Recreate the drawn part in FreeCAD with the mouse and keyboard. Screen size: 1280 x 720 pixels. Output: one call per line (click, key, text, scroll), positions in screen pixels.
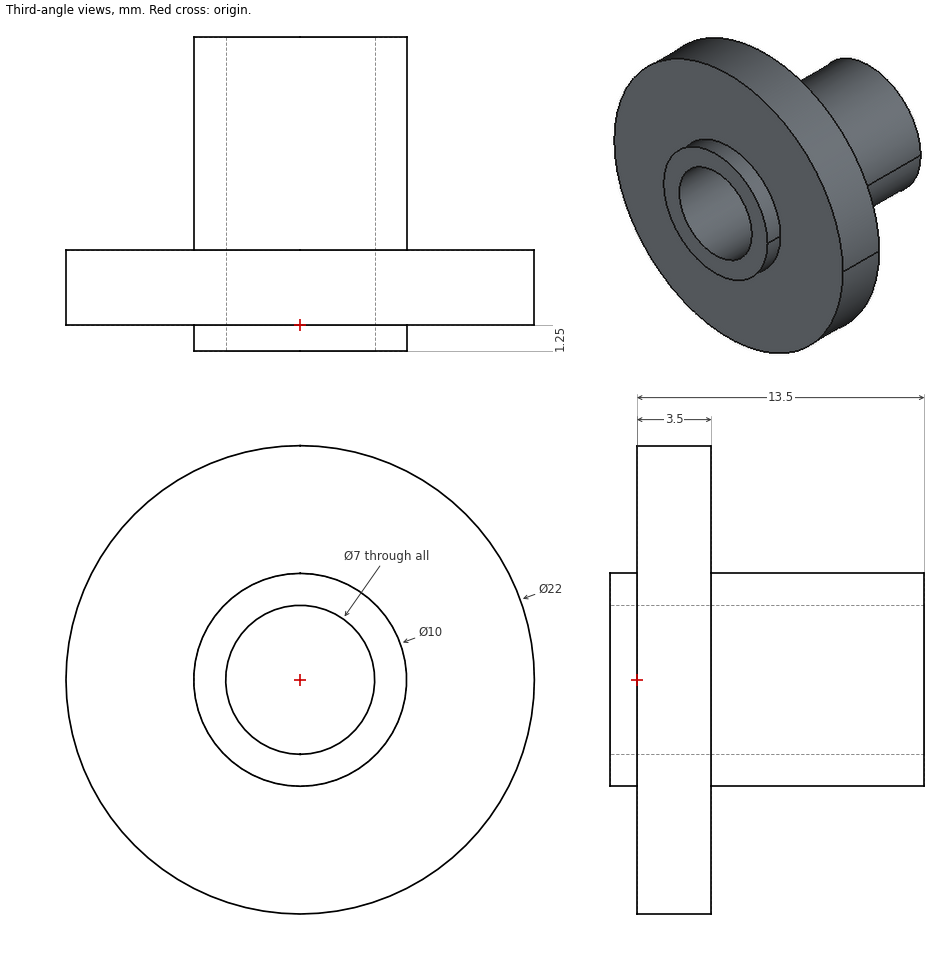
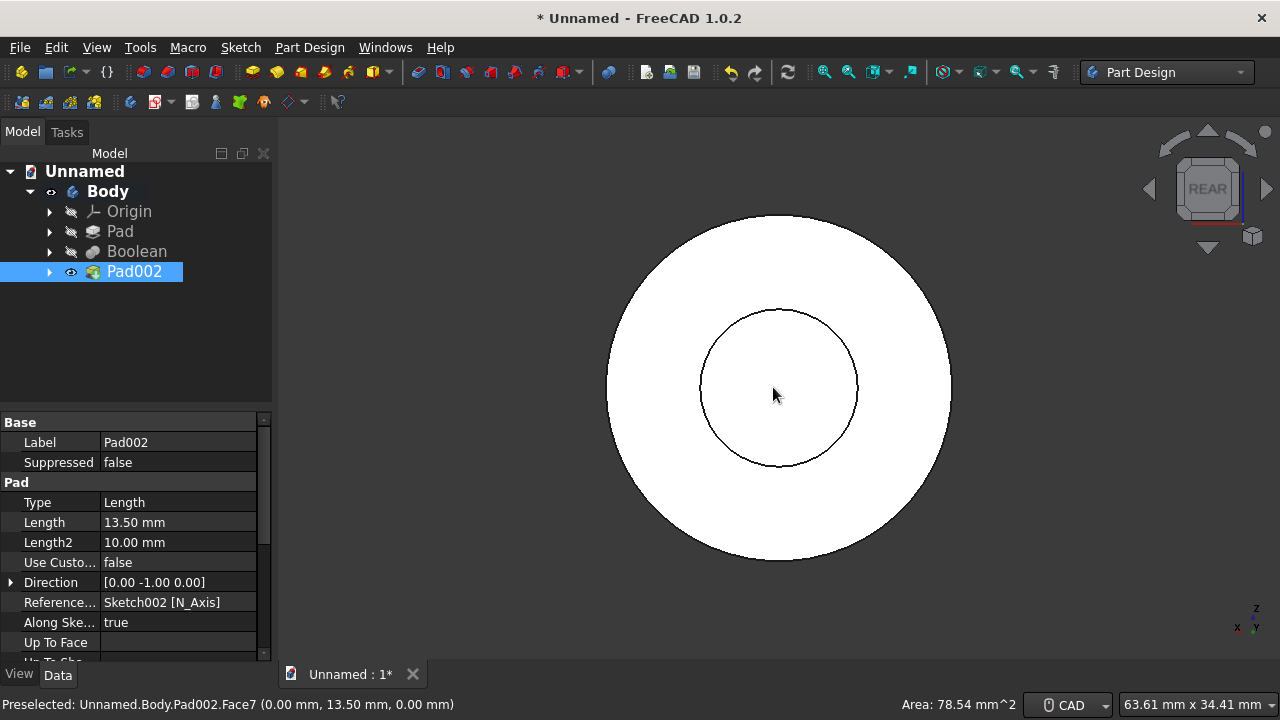
click(156, 102)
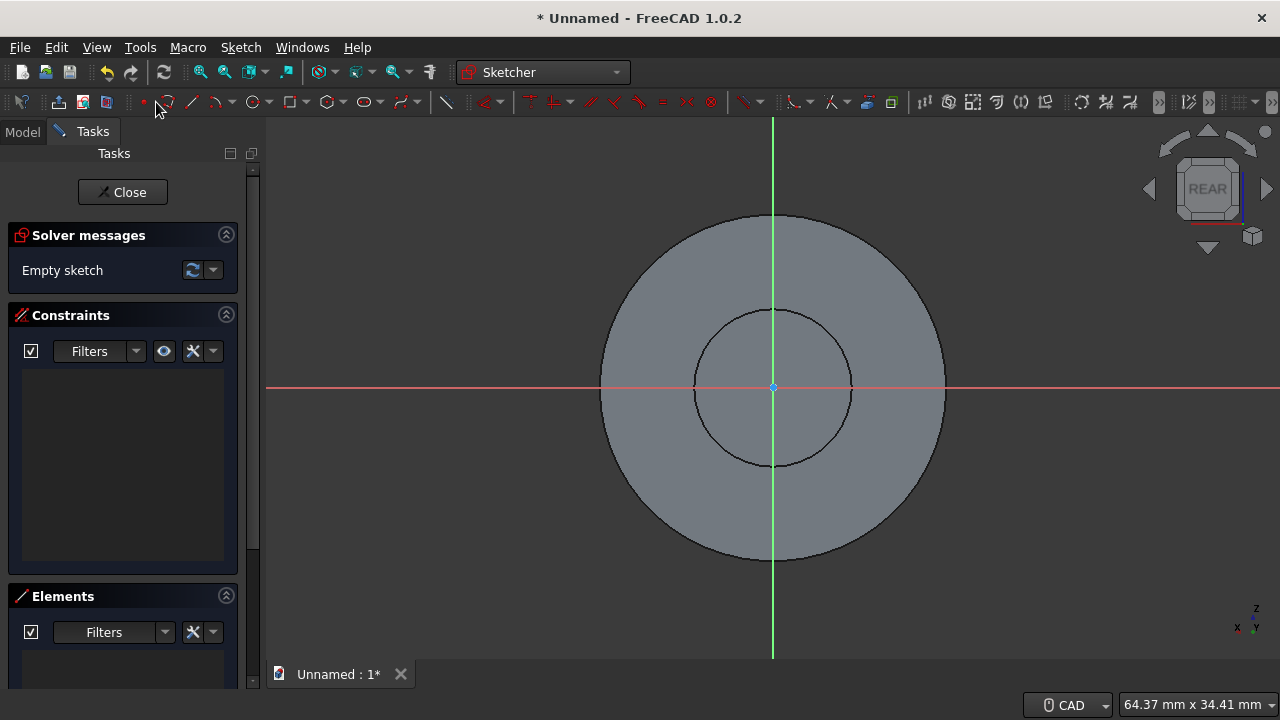
scroll(803, 388, up, 6)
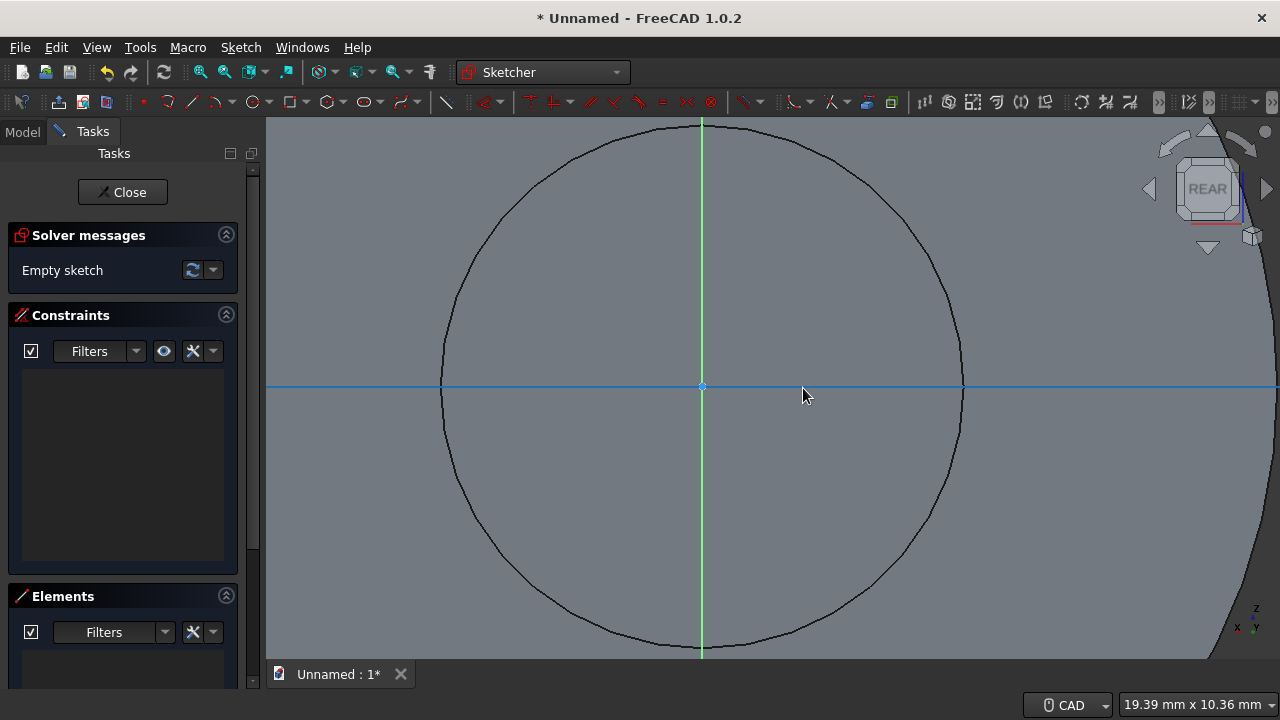
click(254, 102)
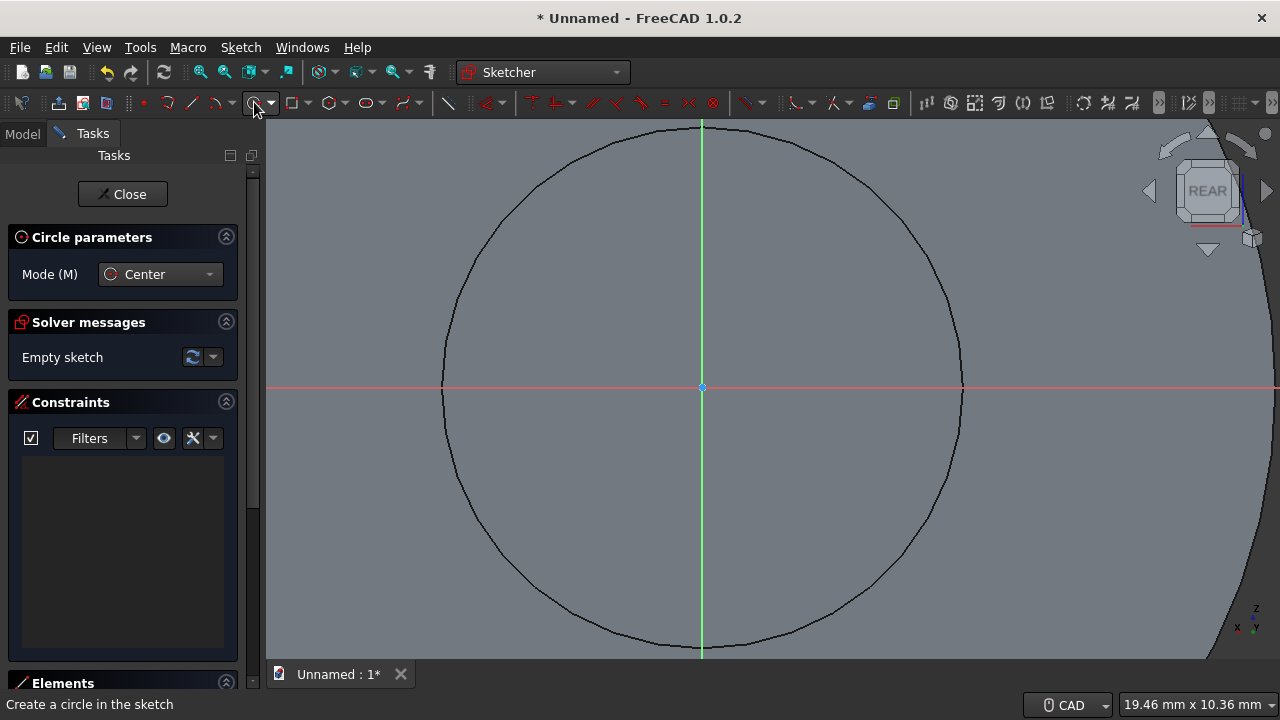
click(702, 388)
move(831, 259)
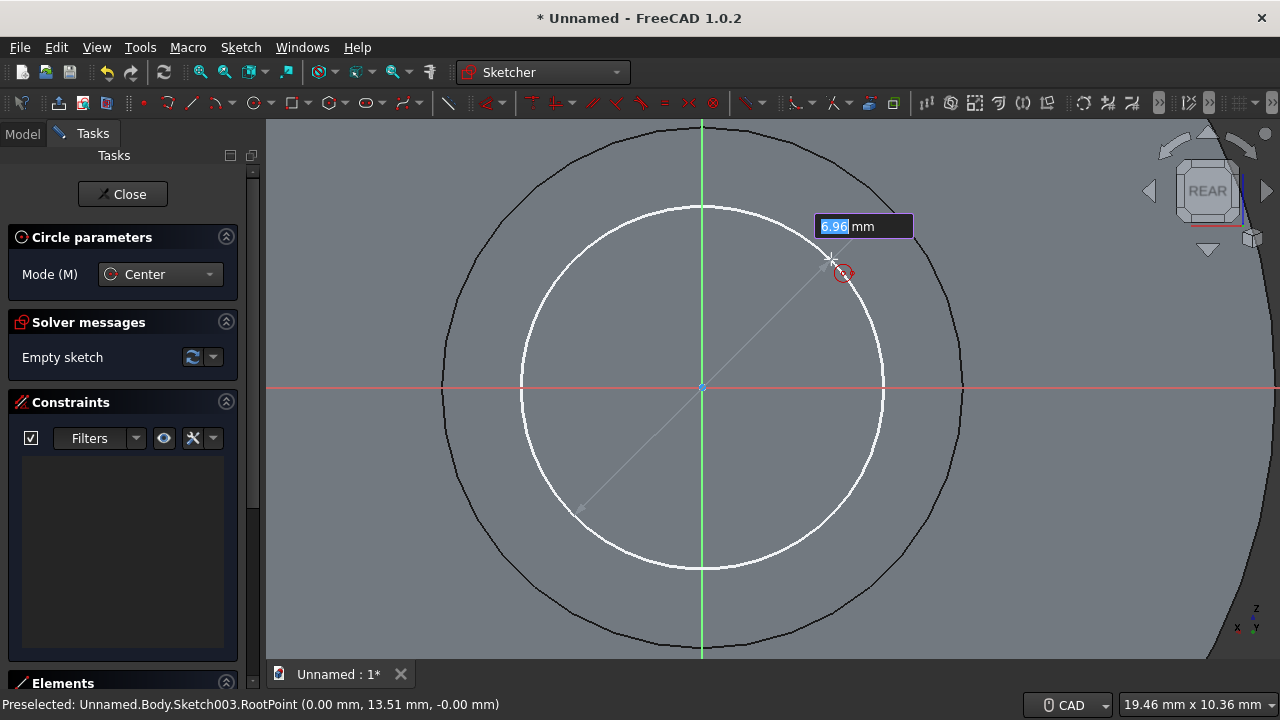
text(7)
key(Return)
key(Escape)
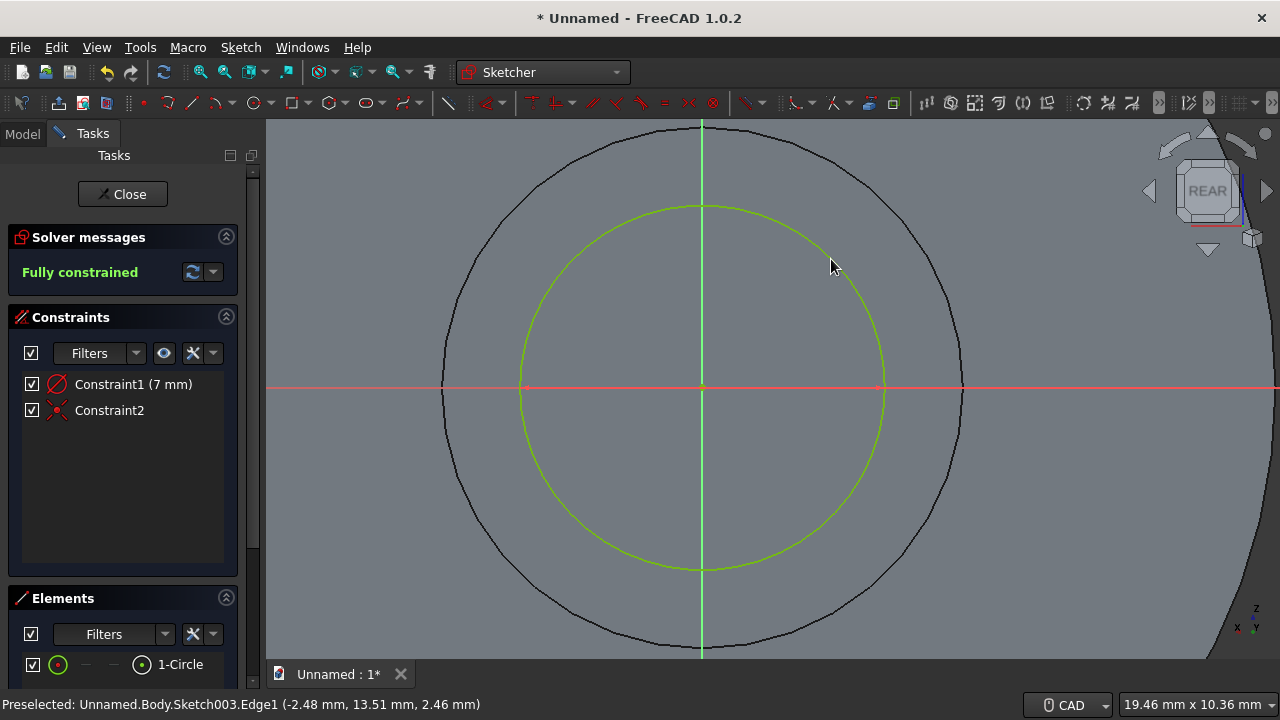
click(123, 194)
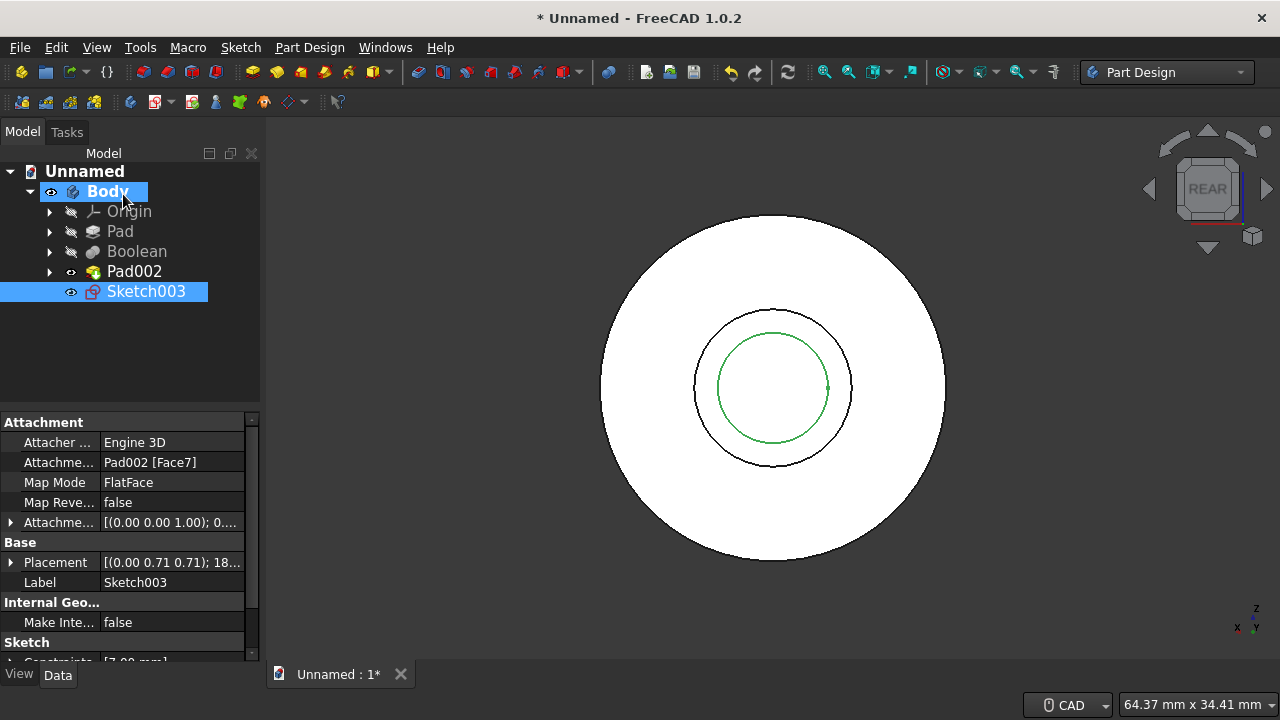
click(444, 72)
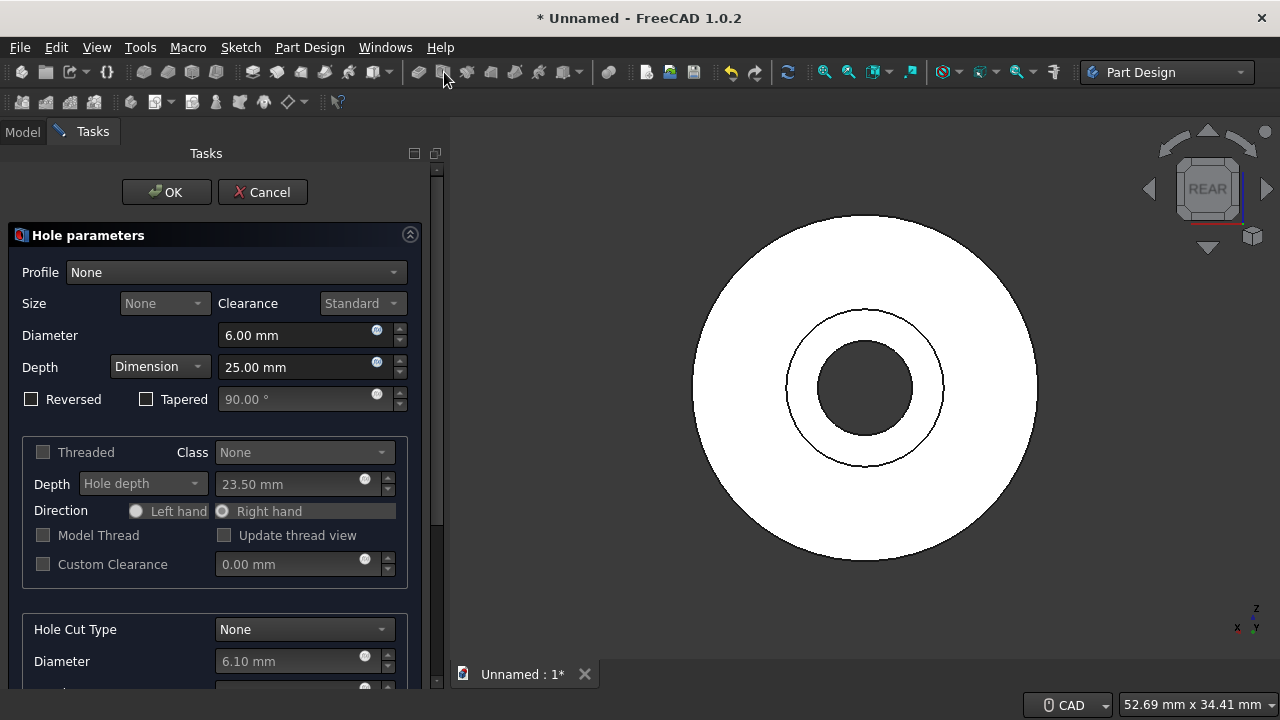
triple_click(305, 335)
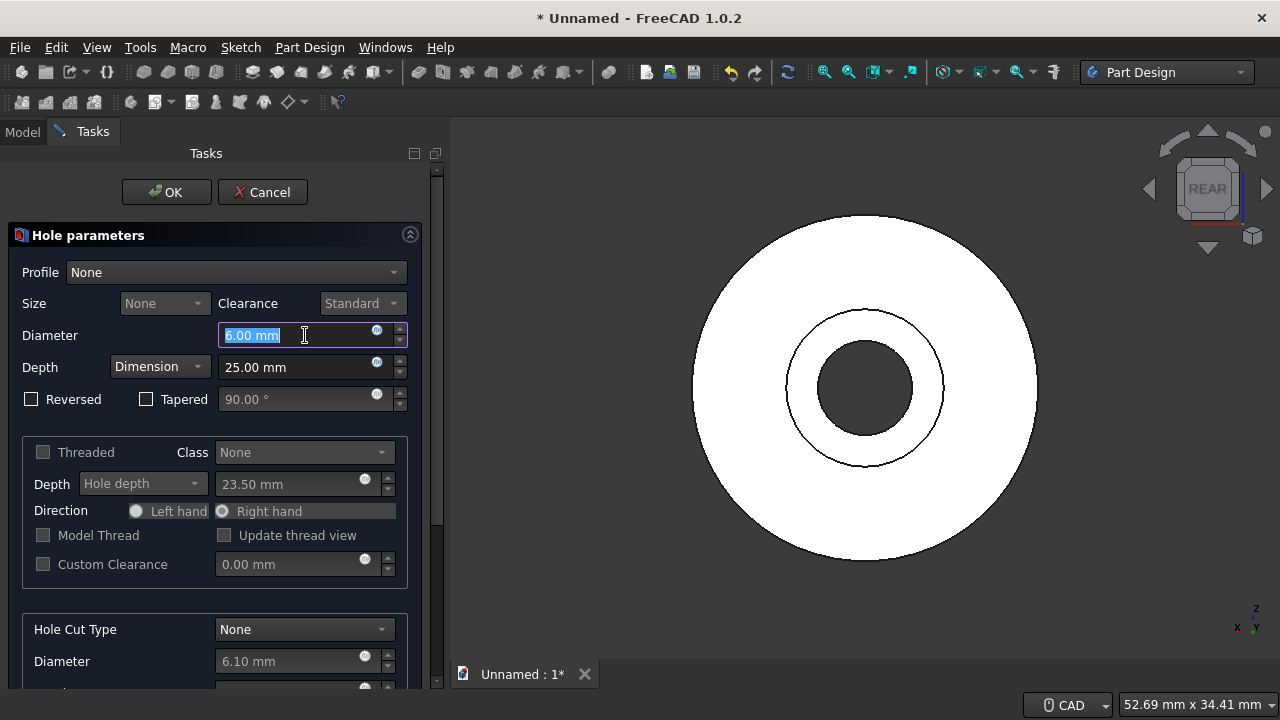
text(7)
key(Tab)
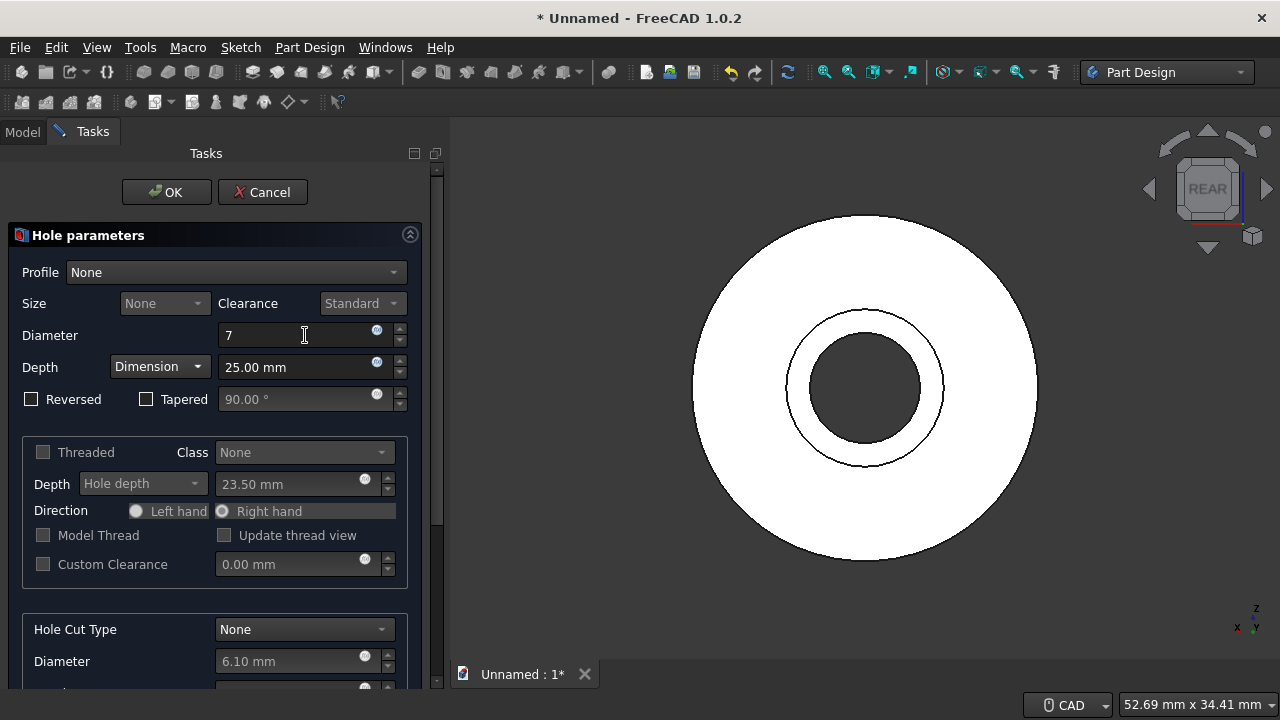
click(161, 366)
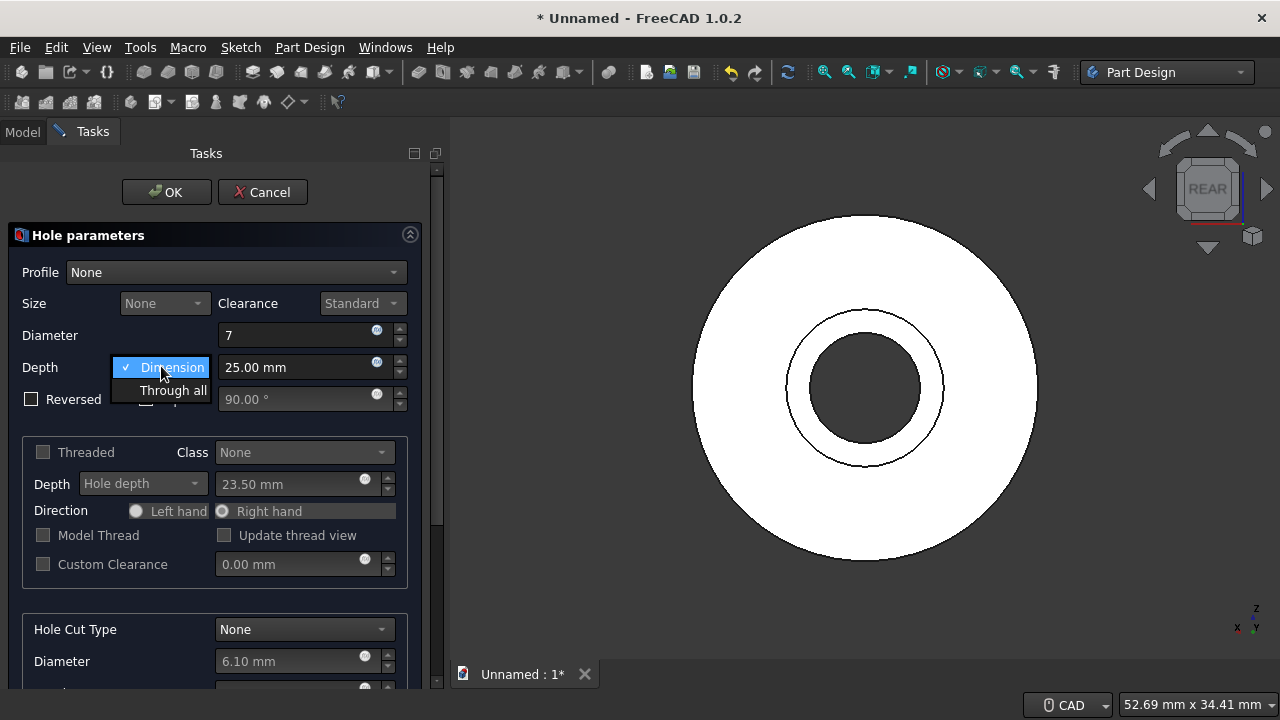
click(160, 390)